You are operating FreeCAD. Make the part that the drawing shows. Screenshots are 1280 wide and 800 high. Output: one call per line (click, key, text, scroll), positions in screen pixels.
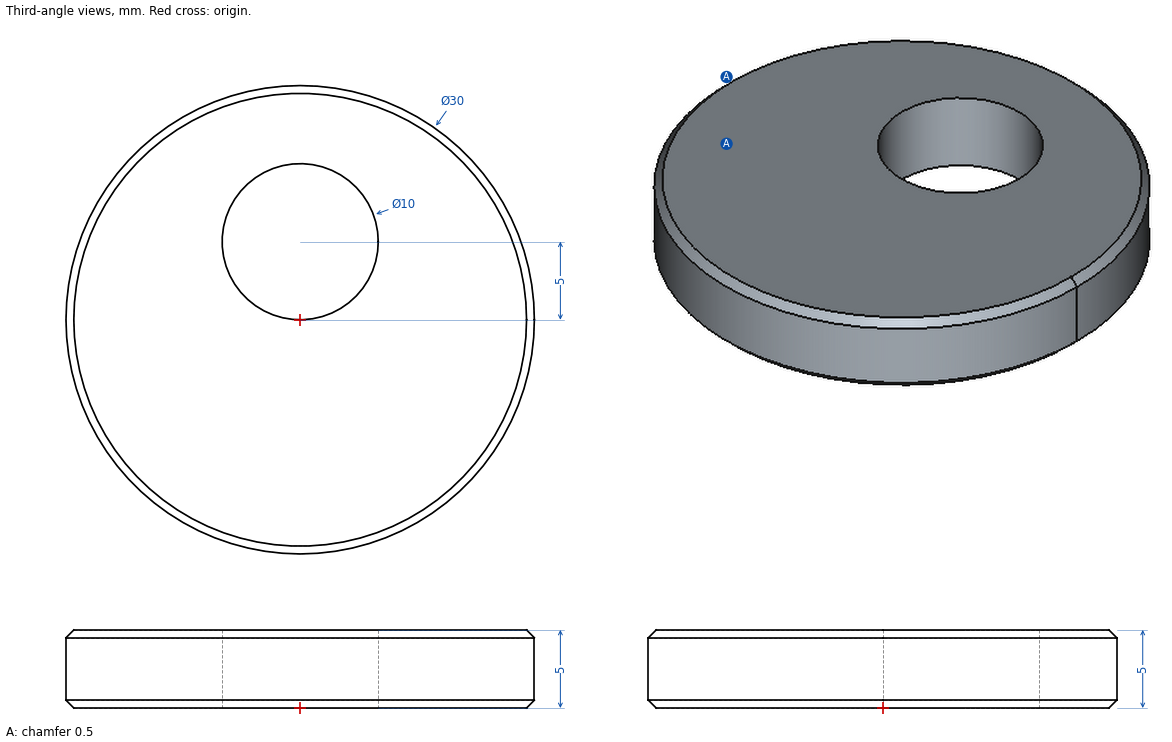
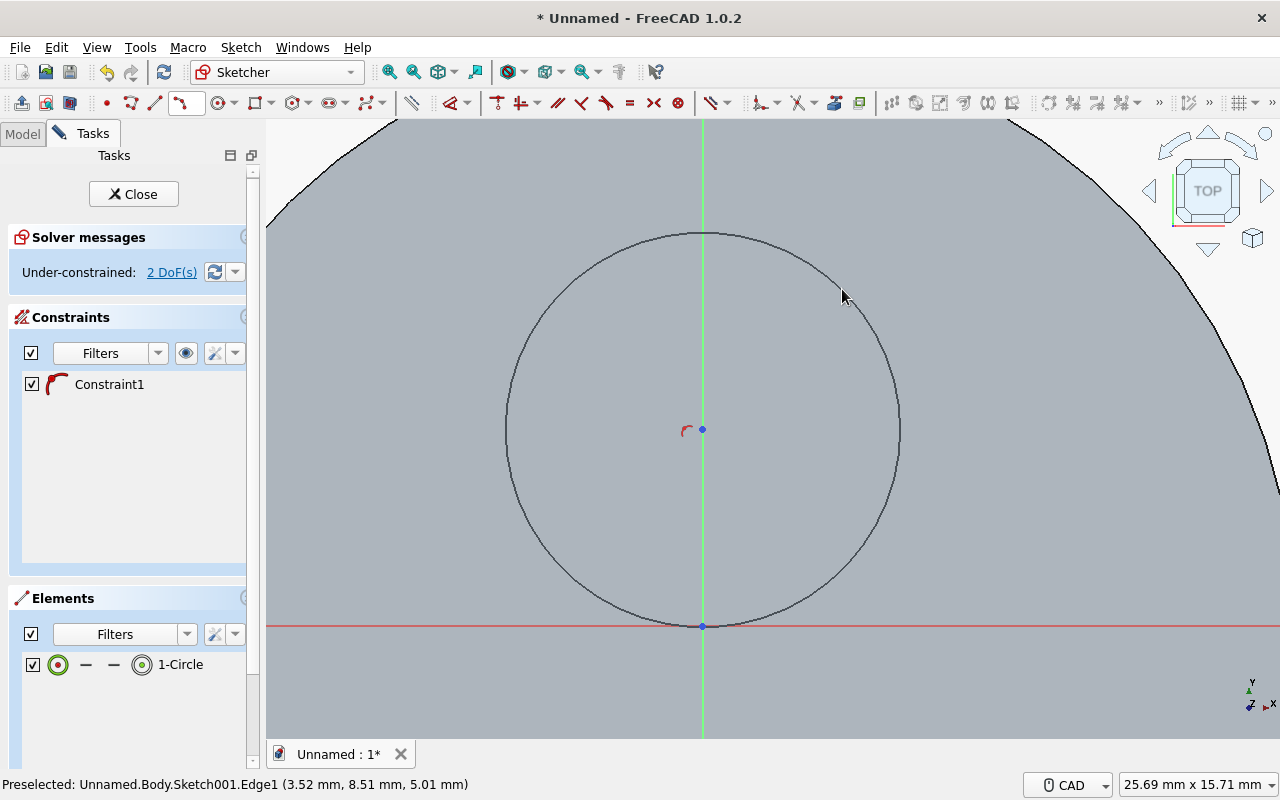
key(d)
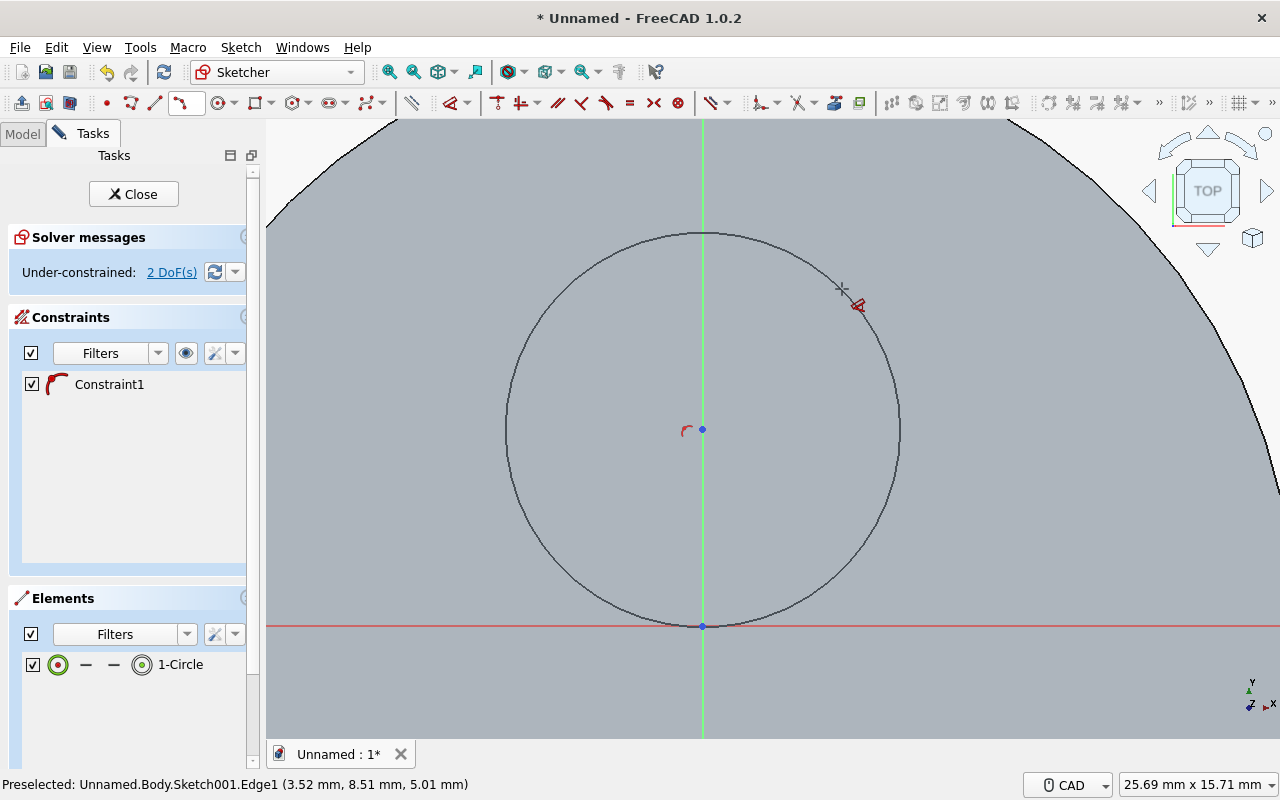
click(842, 290)
click(865, 267)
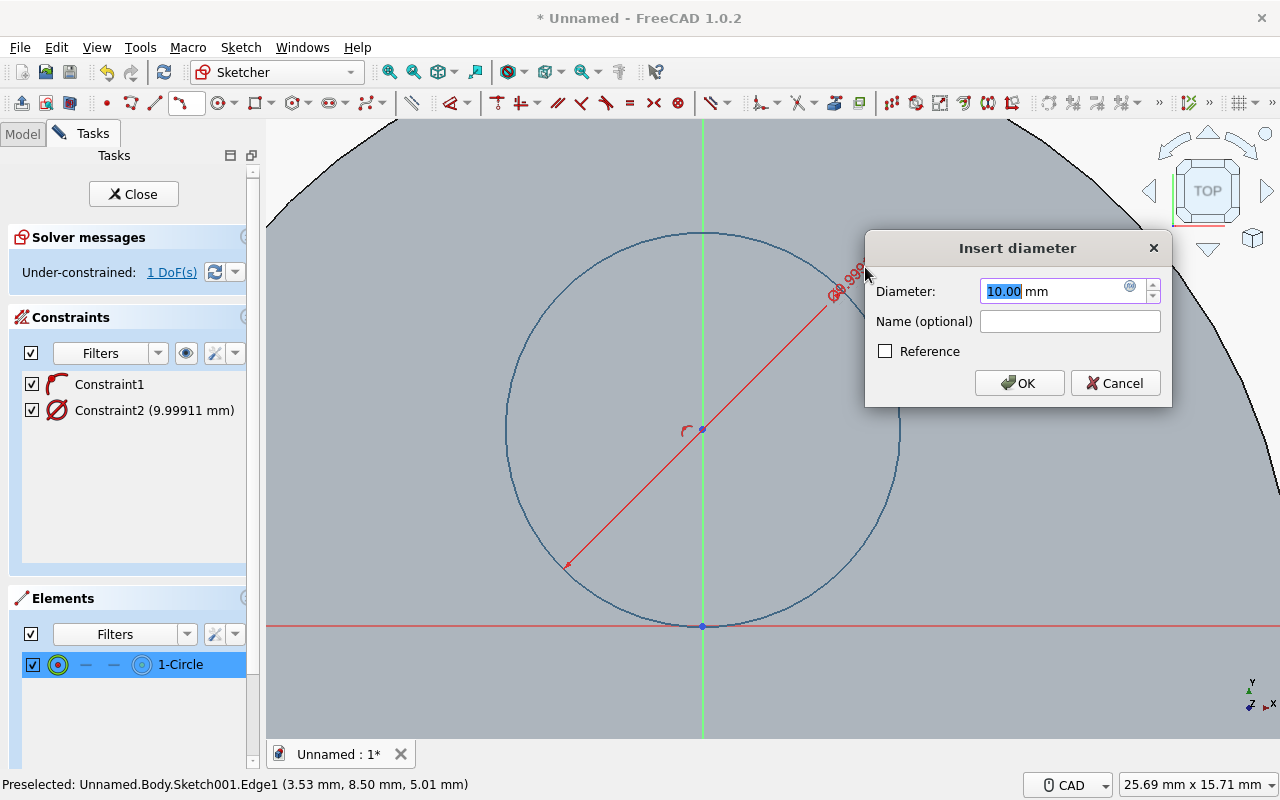
text(10)
key(Return)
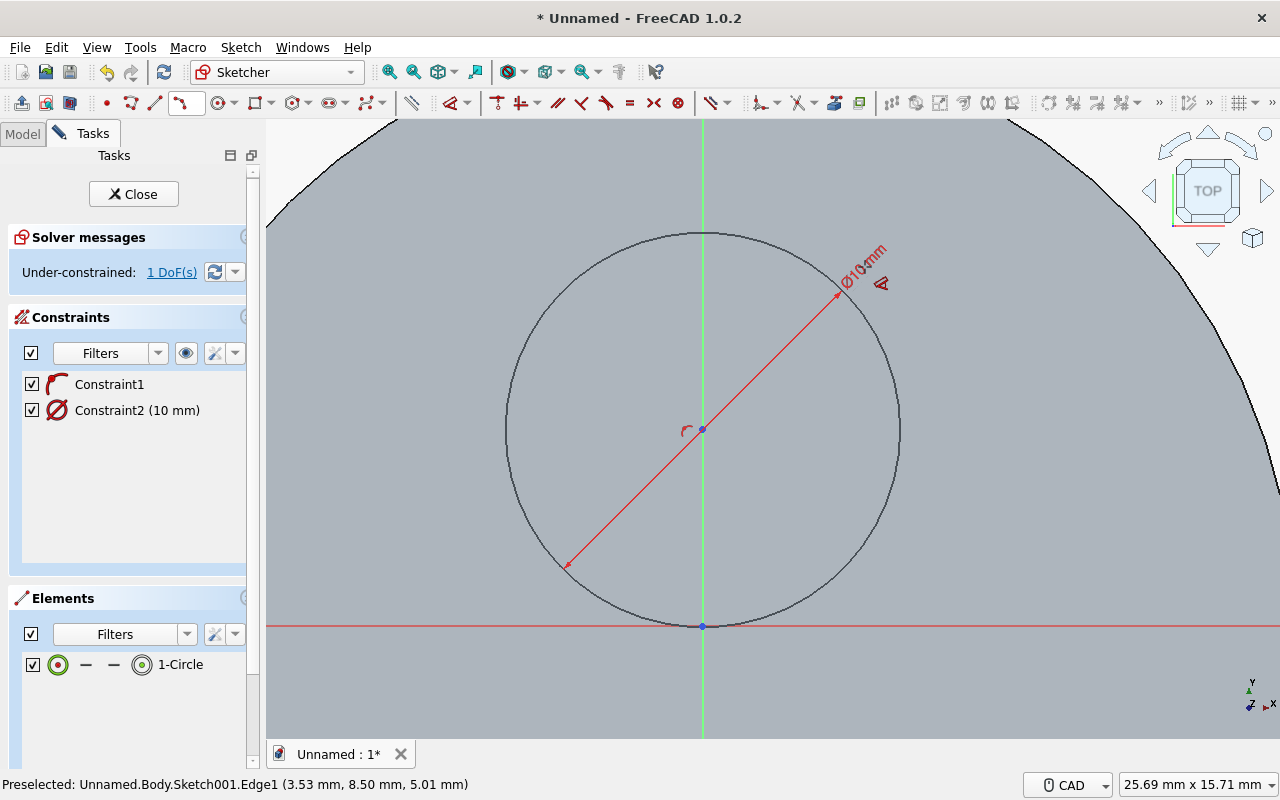
click(703, 430)
click(737, 528)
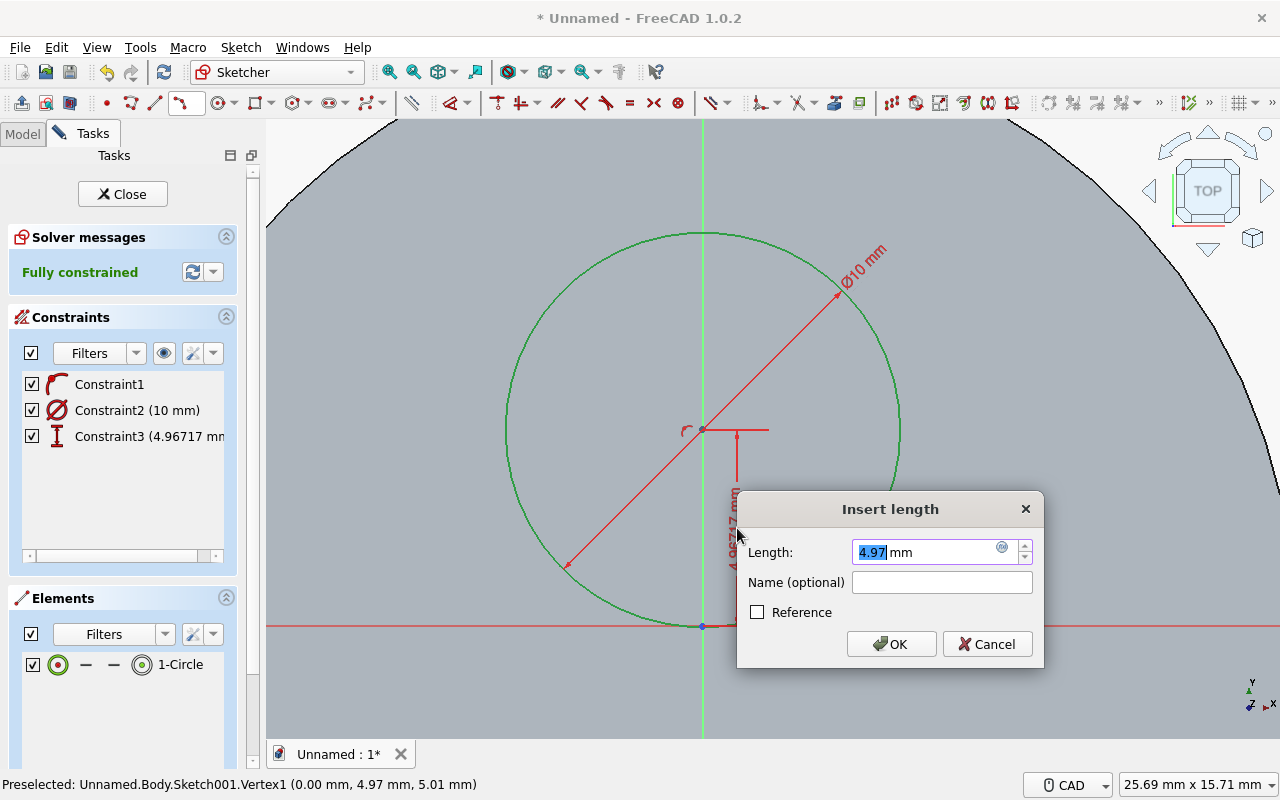
text(5)
key(Return)
key(Escape)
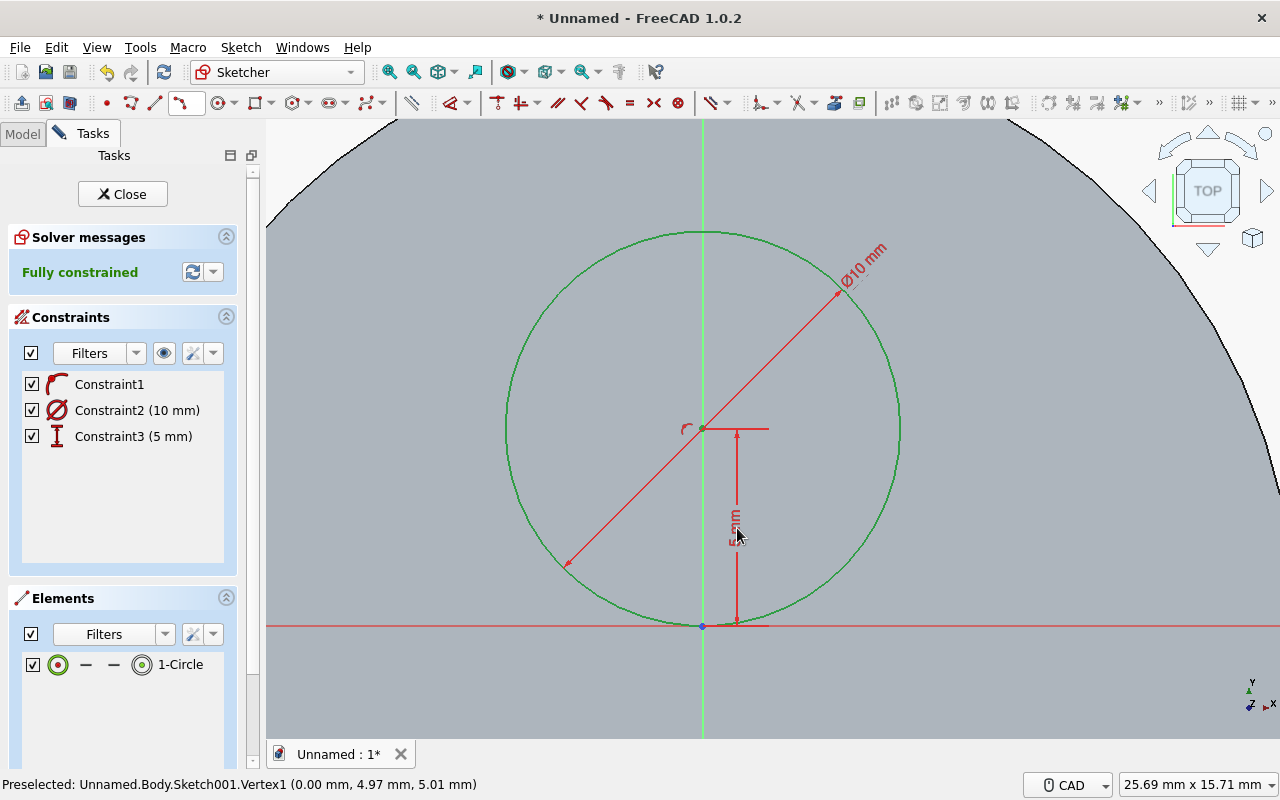
click(123, 194)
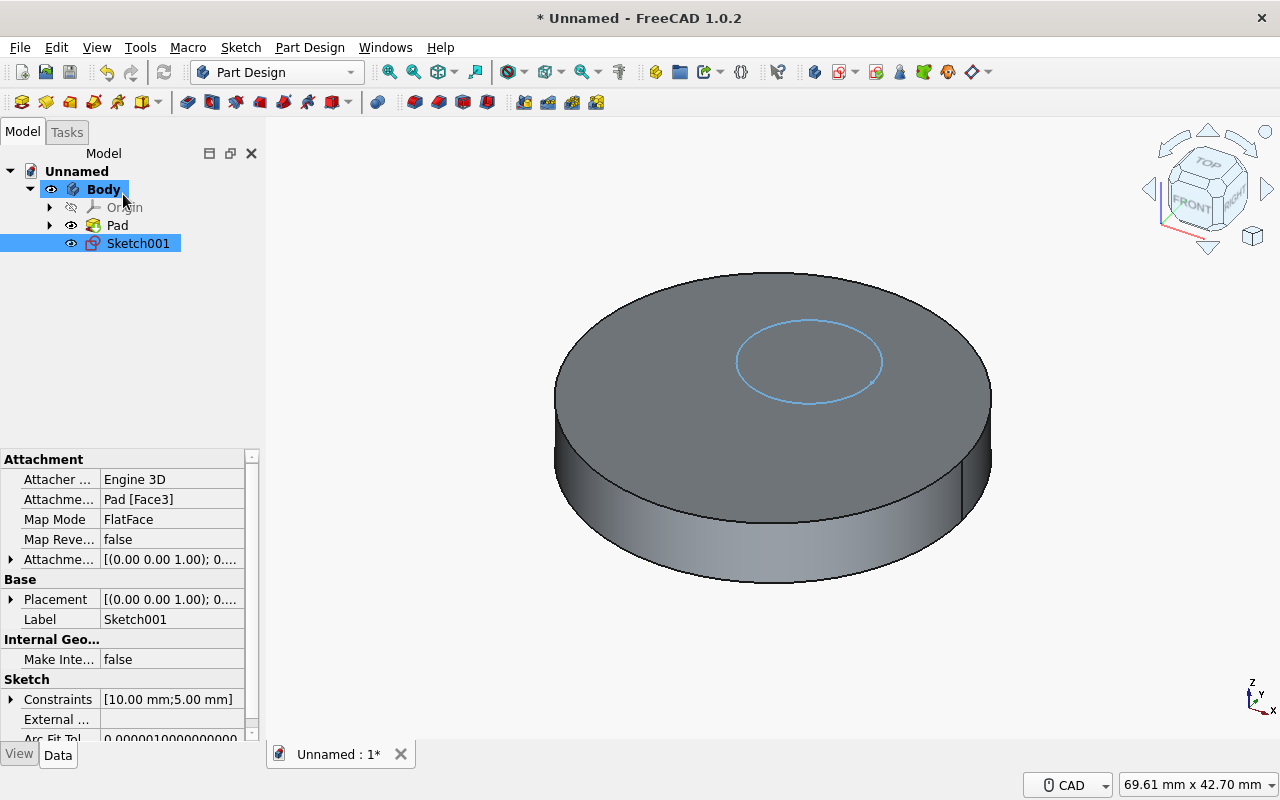
click(188, 102)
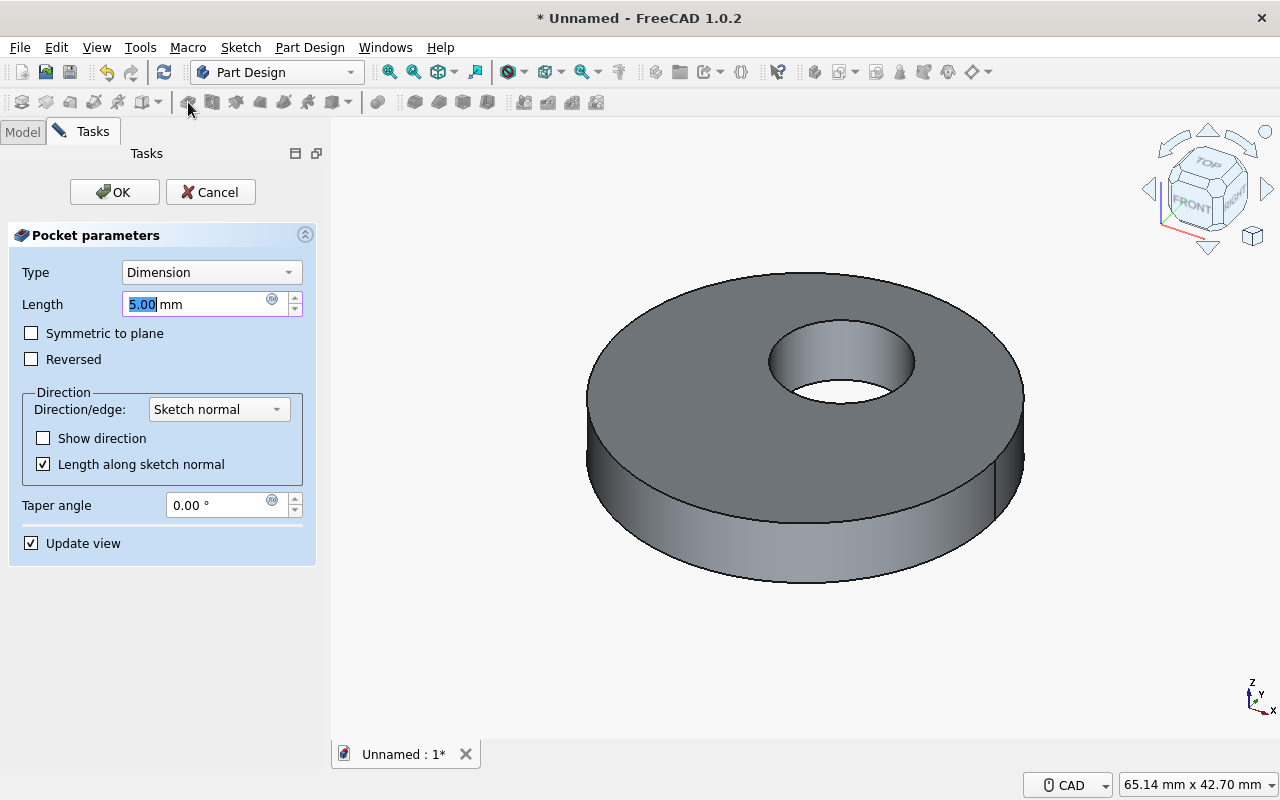
text(5)
key(Tab)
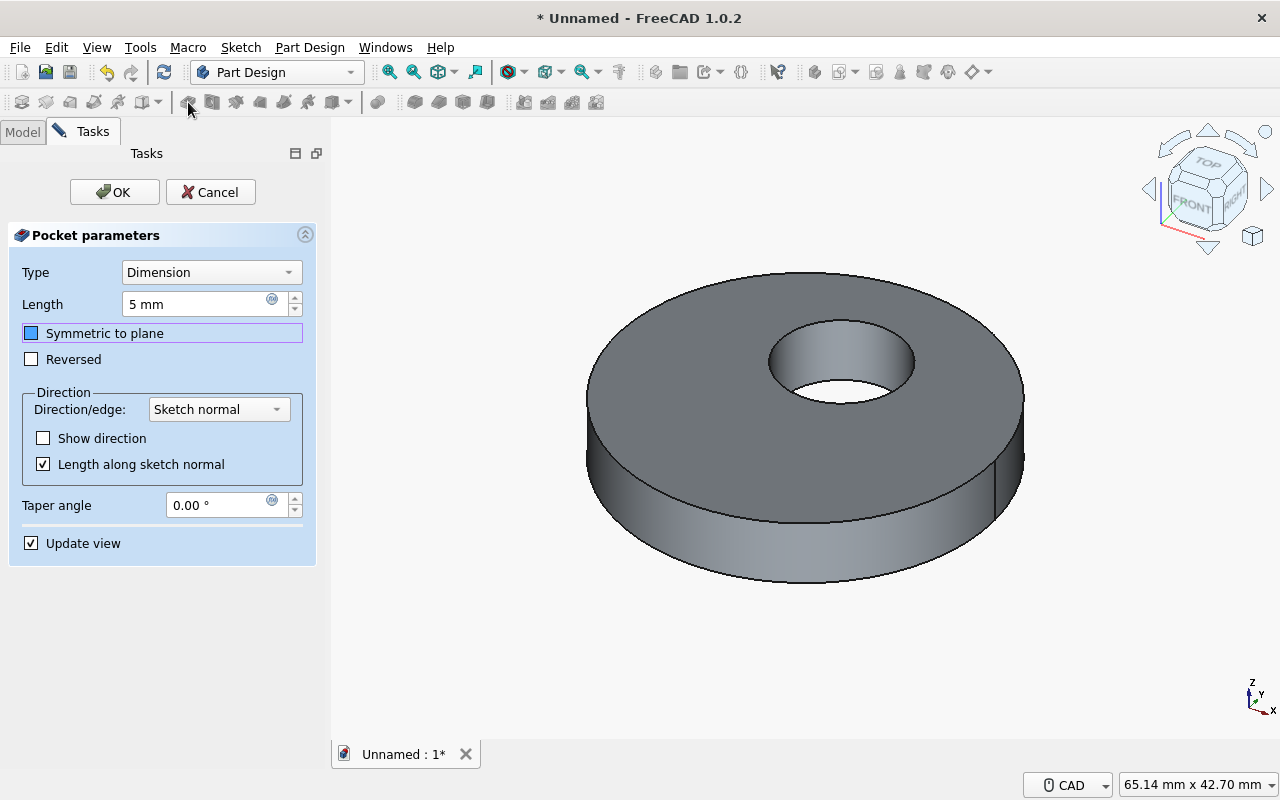
click(115, 192)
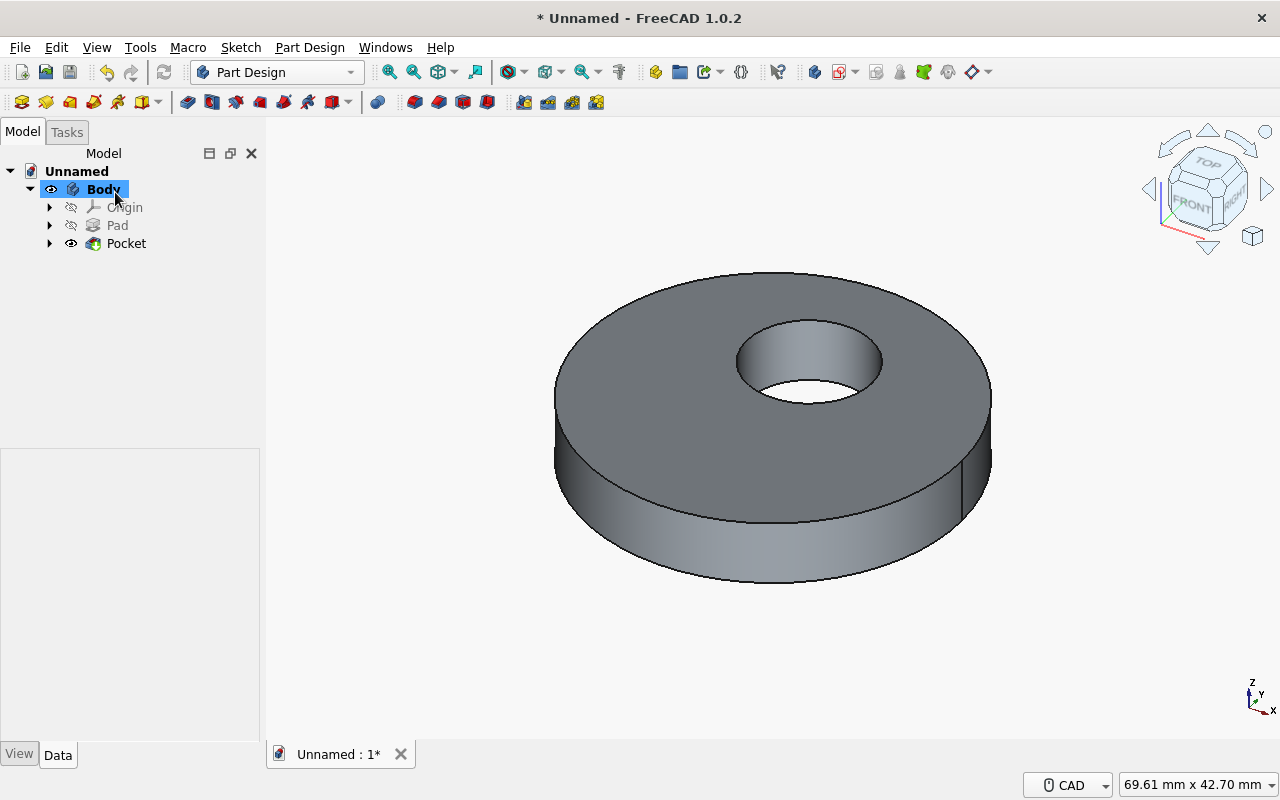
click(556, 410)